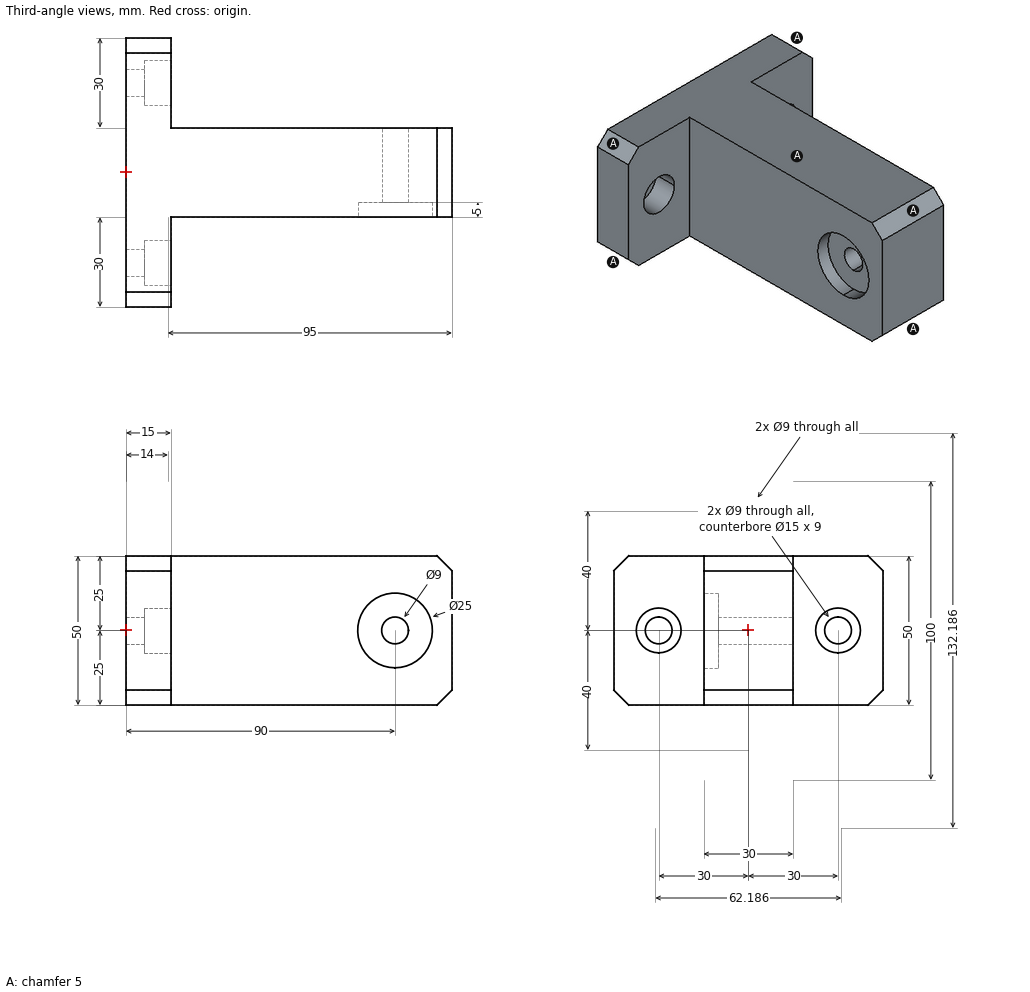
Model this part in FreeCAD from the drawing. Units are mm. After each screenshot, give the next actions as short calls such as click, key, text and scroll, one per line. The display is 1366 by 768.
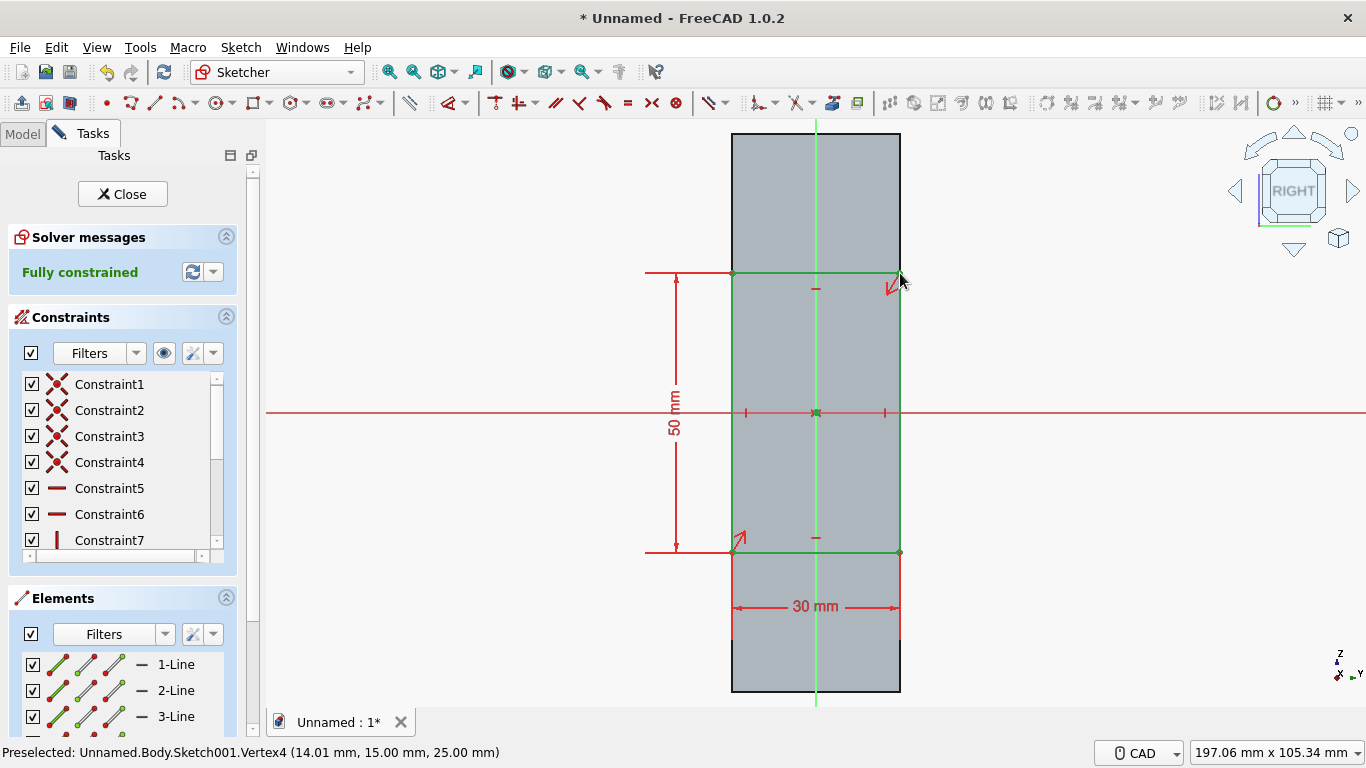
click(123, 194)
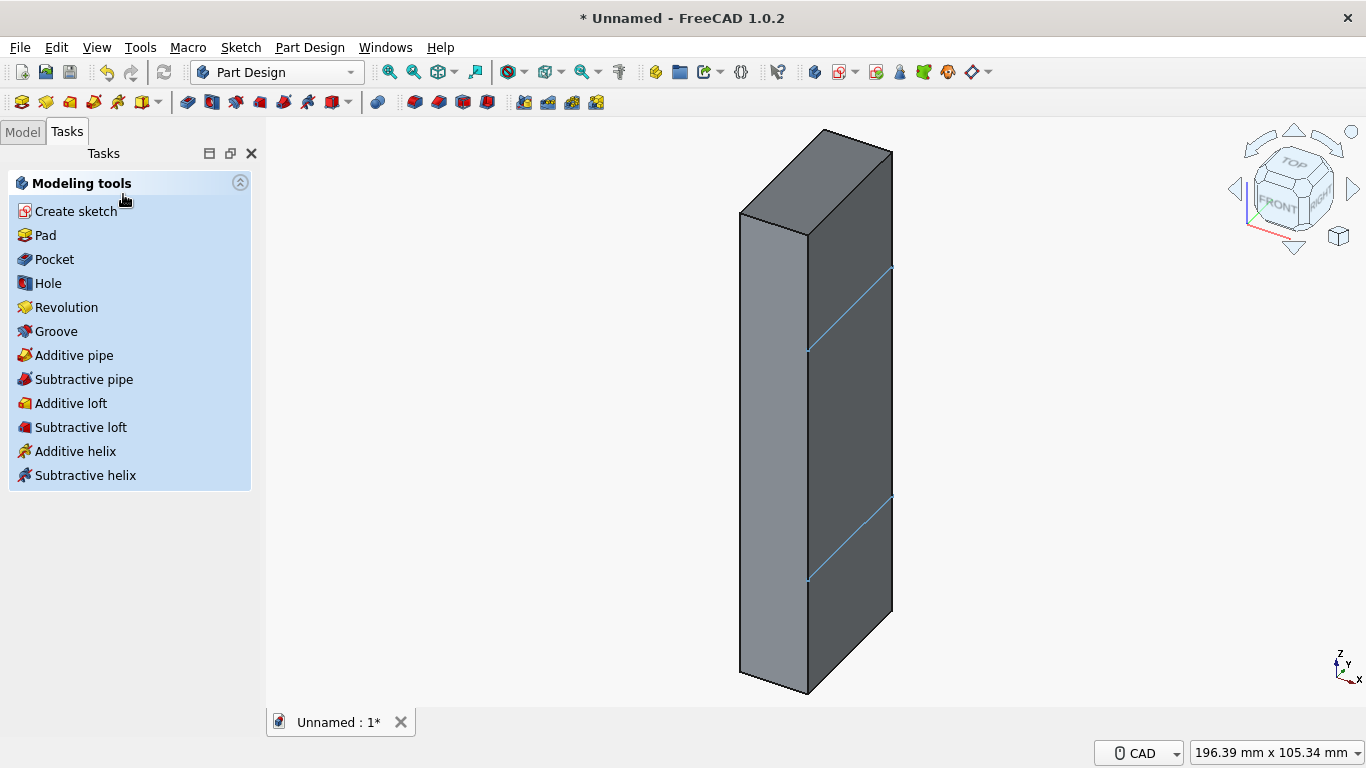
click(22, 102)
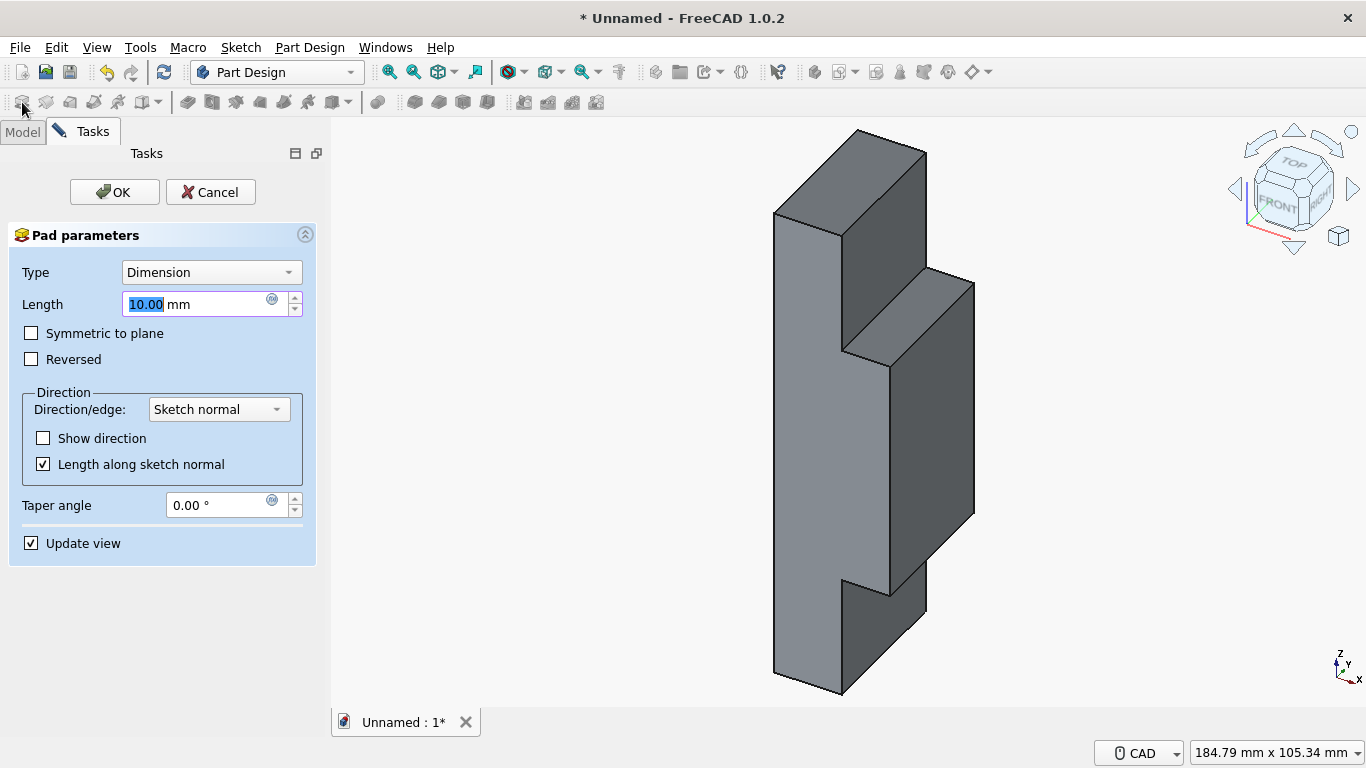
text(95)
key(Tab)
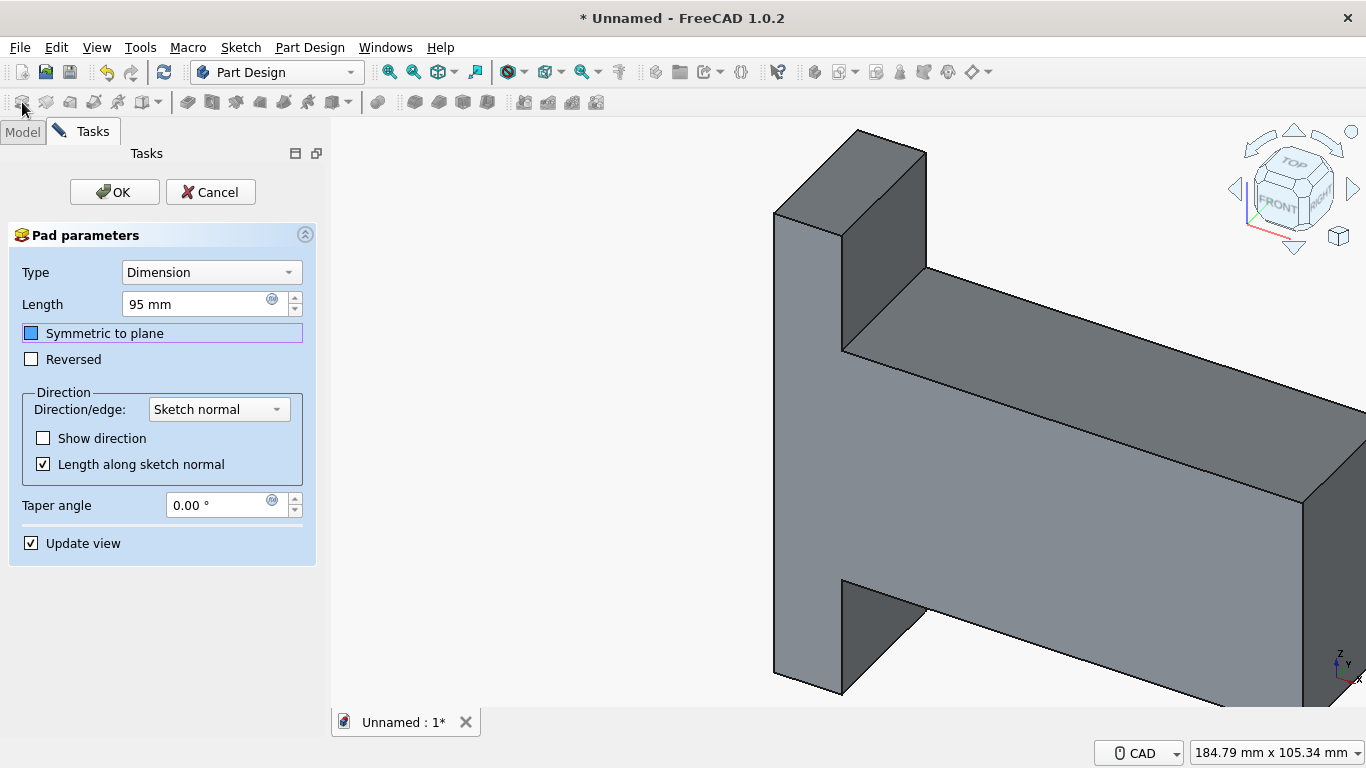
click(115, 192)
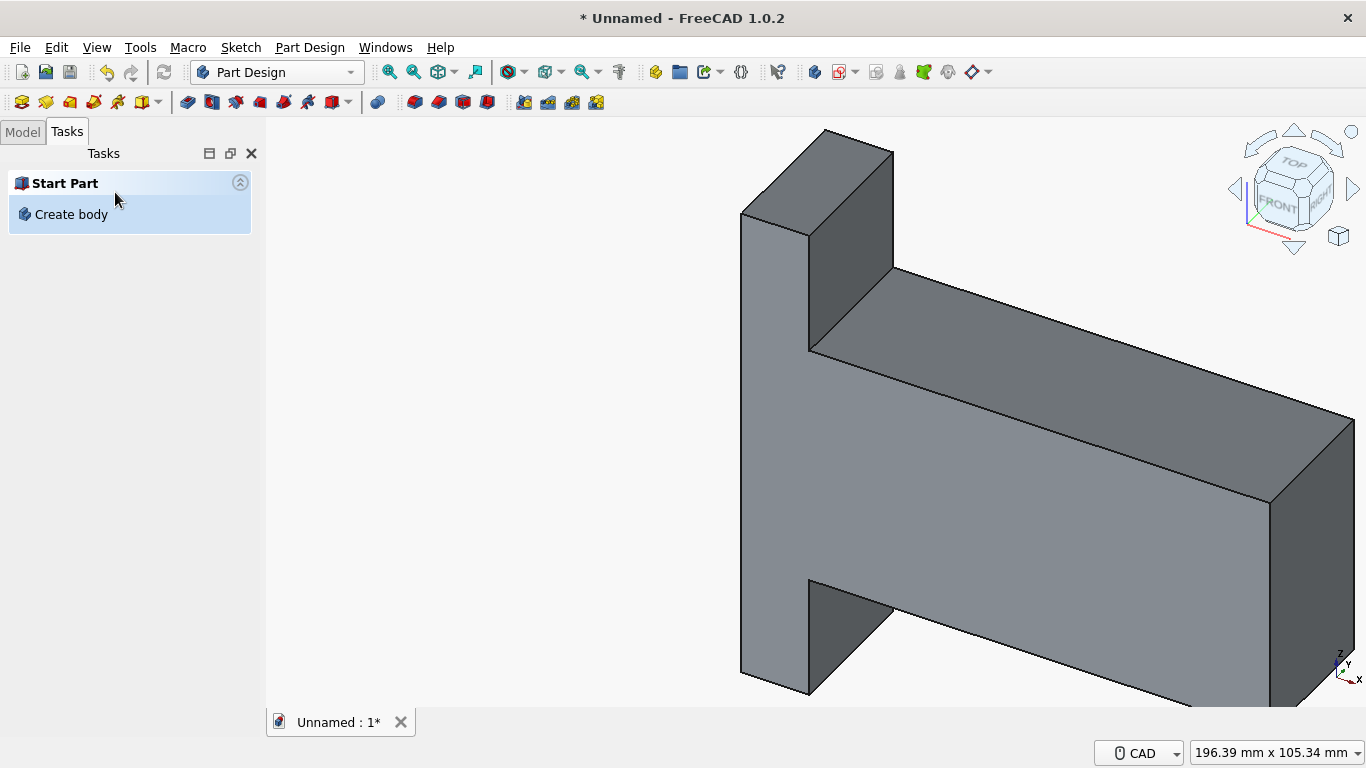
click(390, 72)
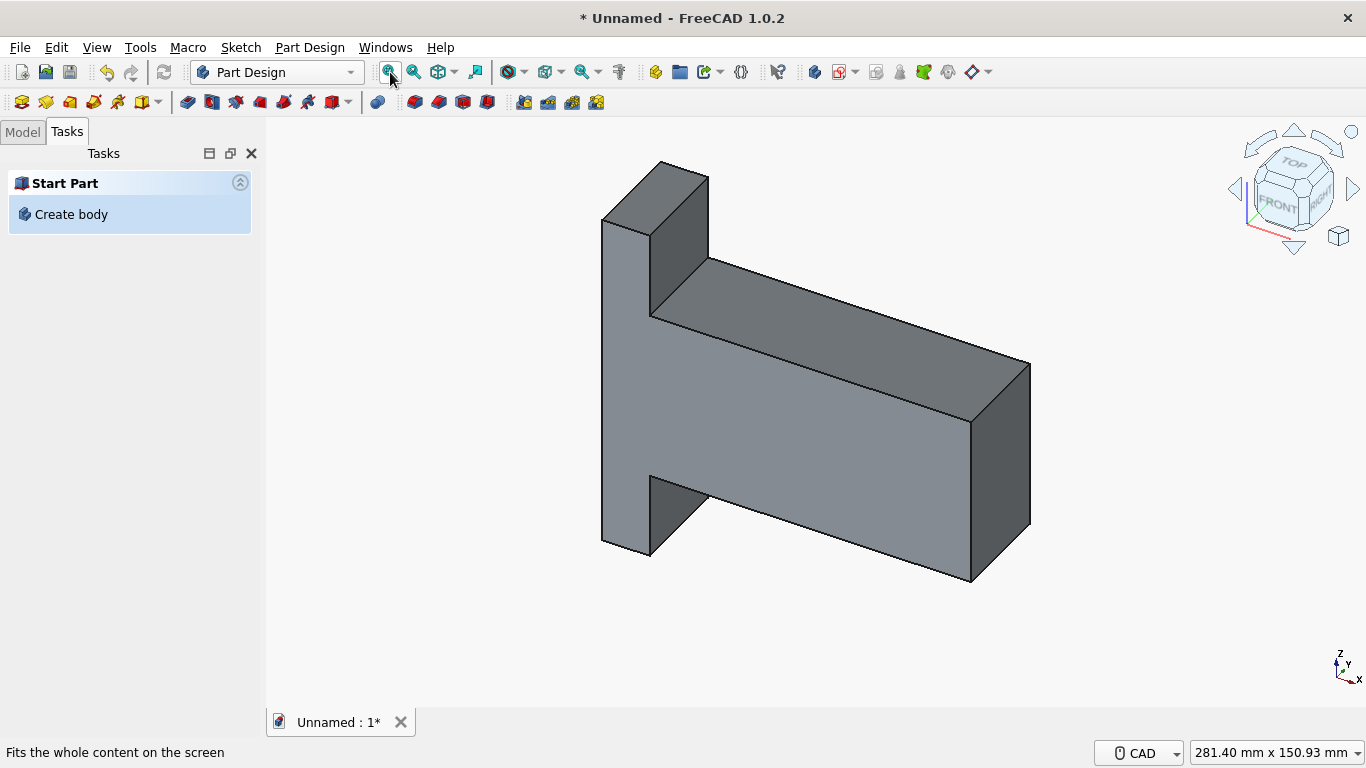
click(839, 458)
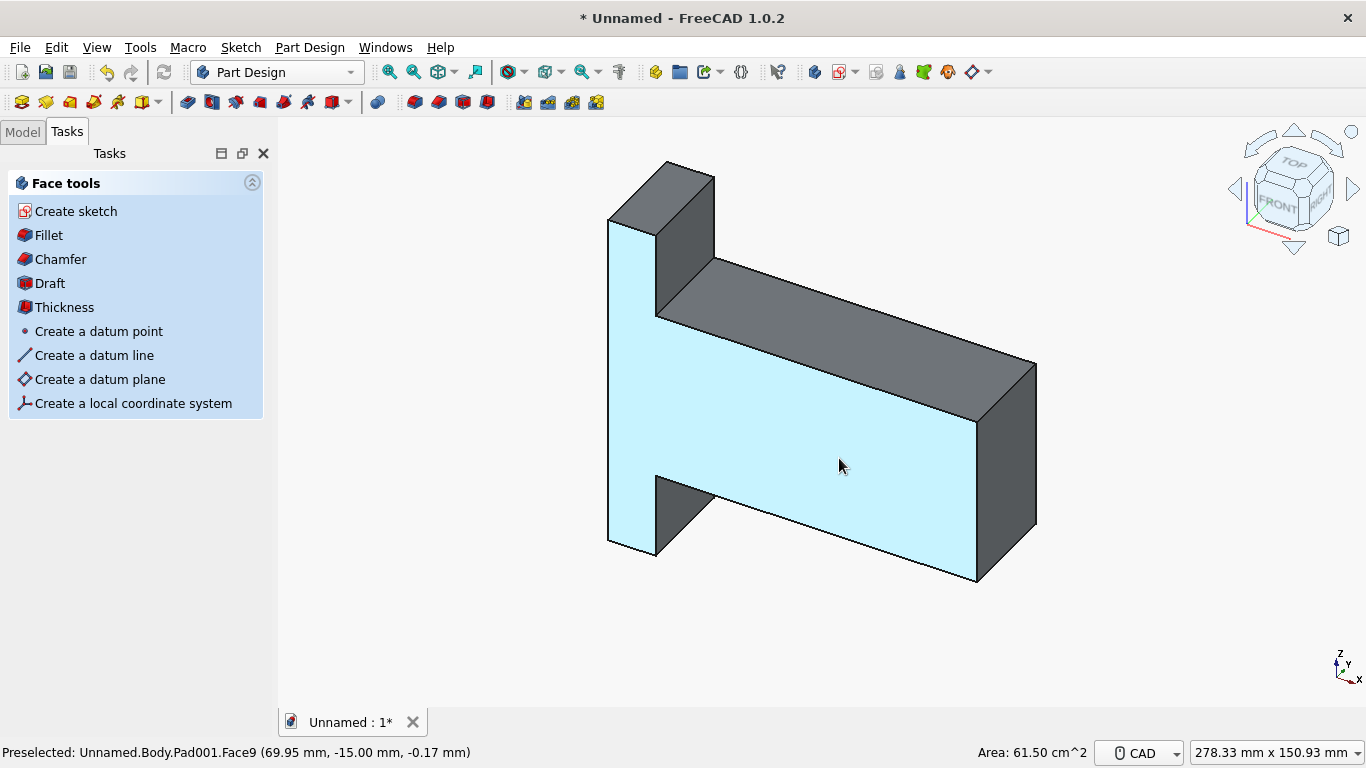
click(840, 72)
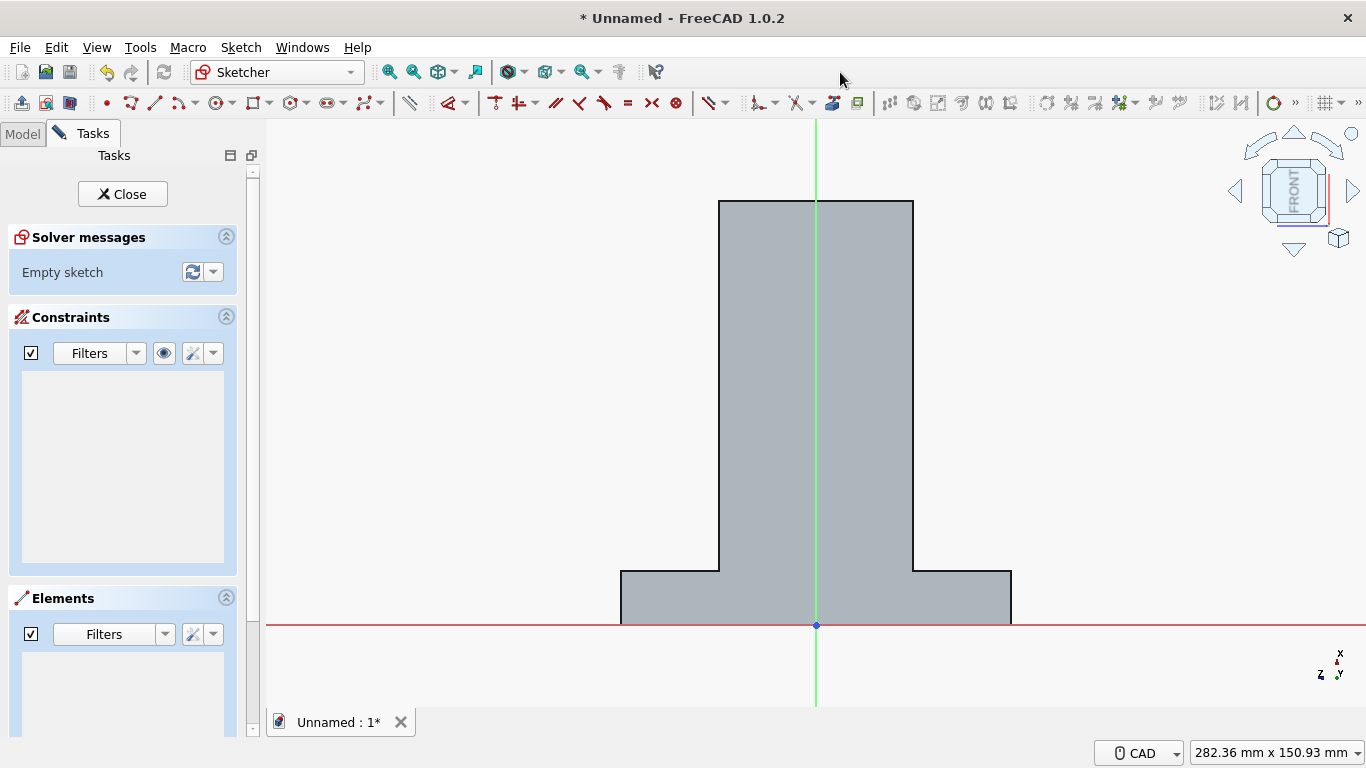
scroll(838, 229, up, 7)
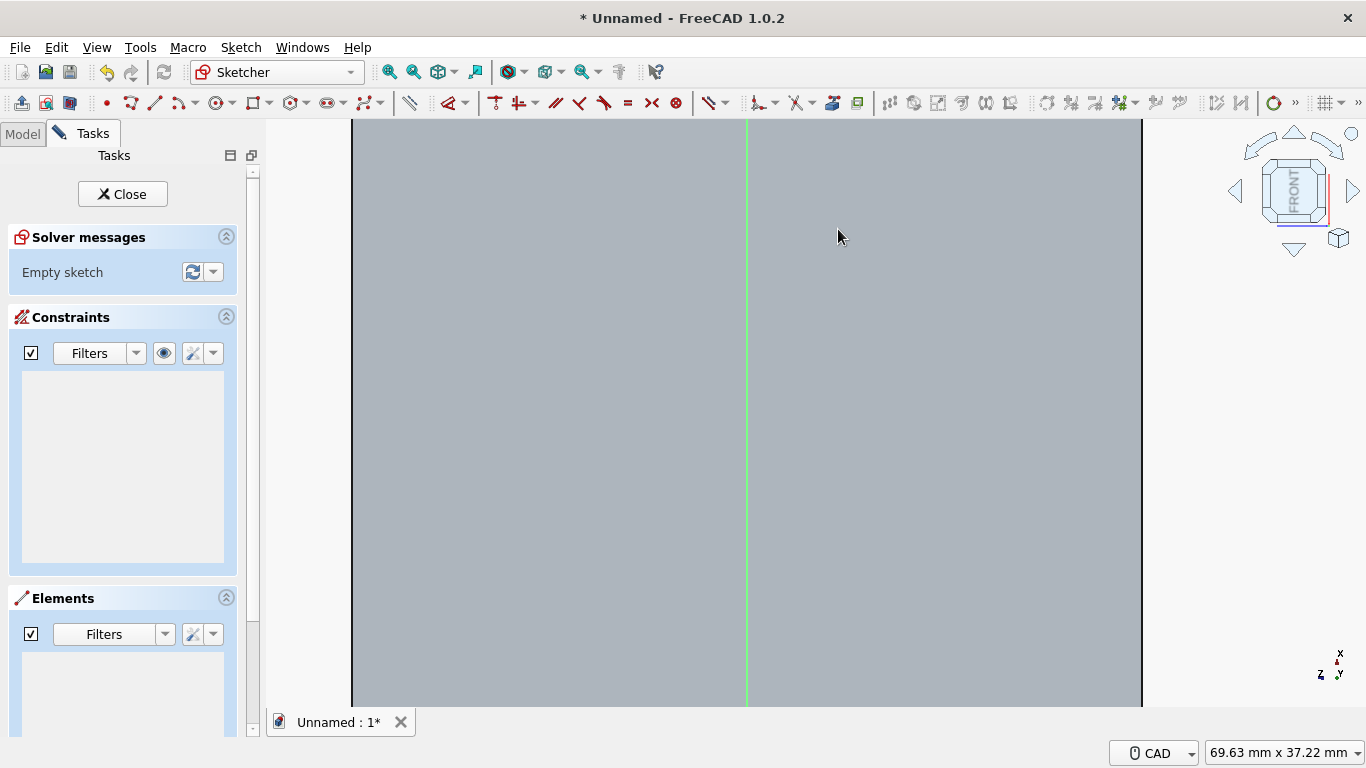
click(216, 104)